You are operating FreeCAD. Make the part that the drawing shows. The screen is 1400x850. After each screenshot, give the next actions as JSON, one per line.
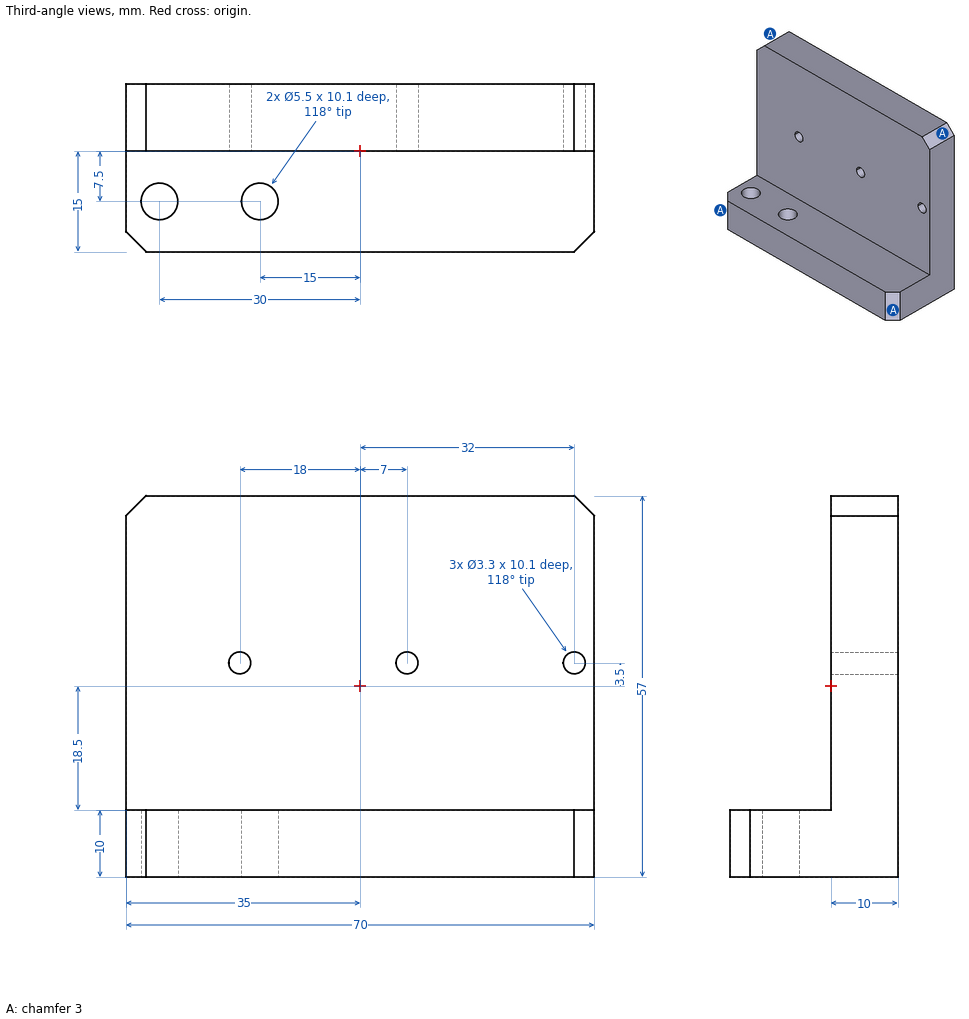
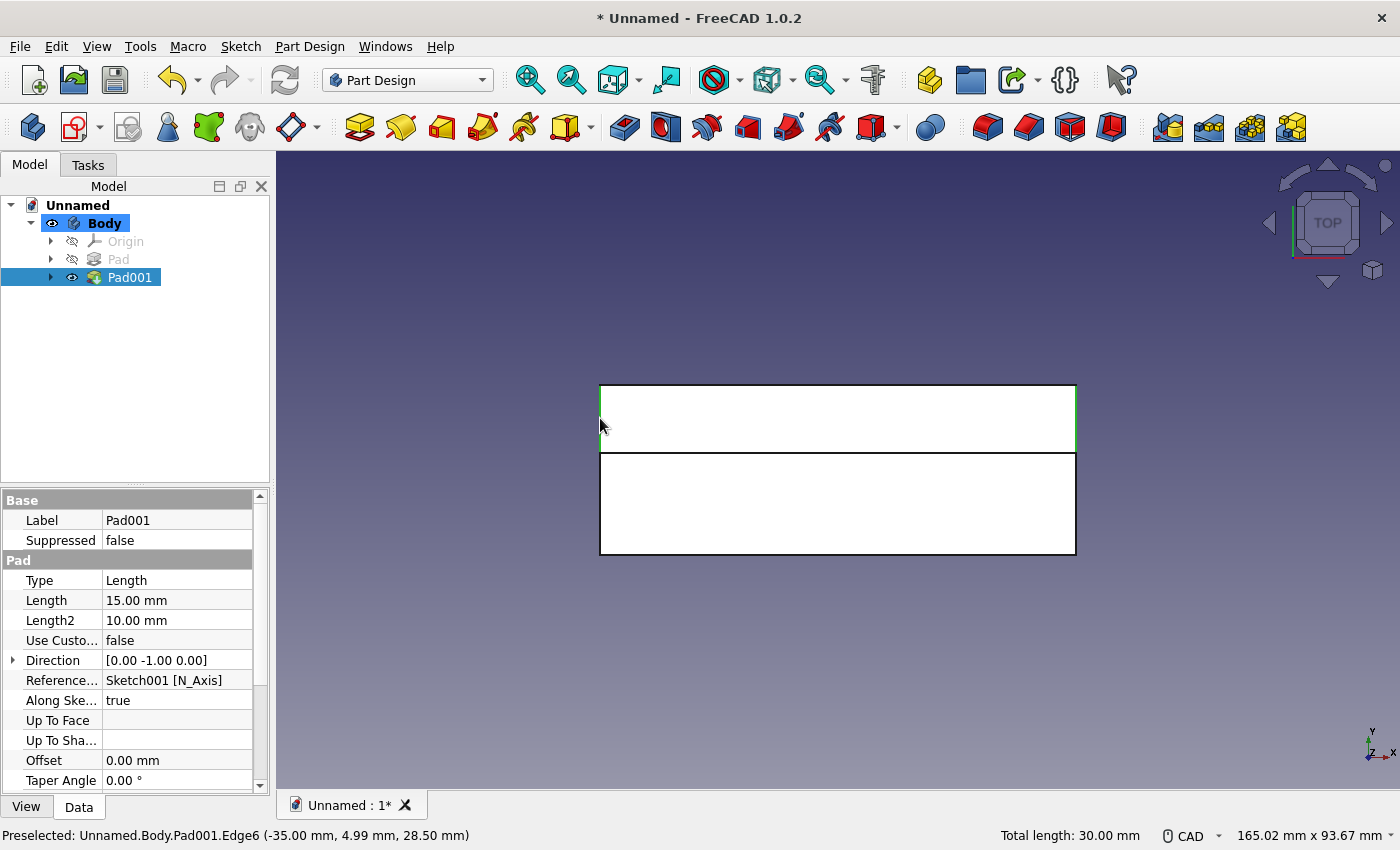
{"action": "key", "text": "1"}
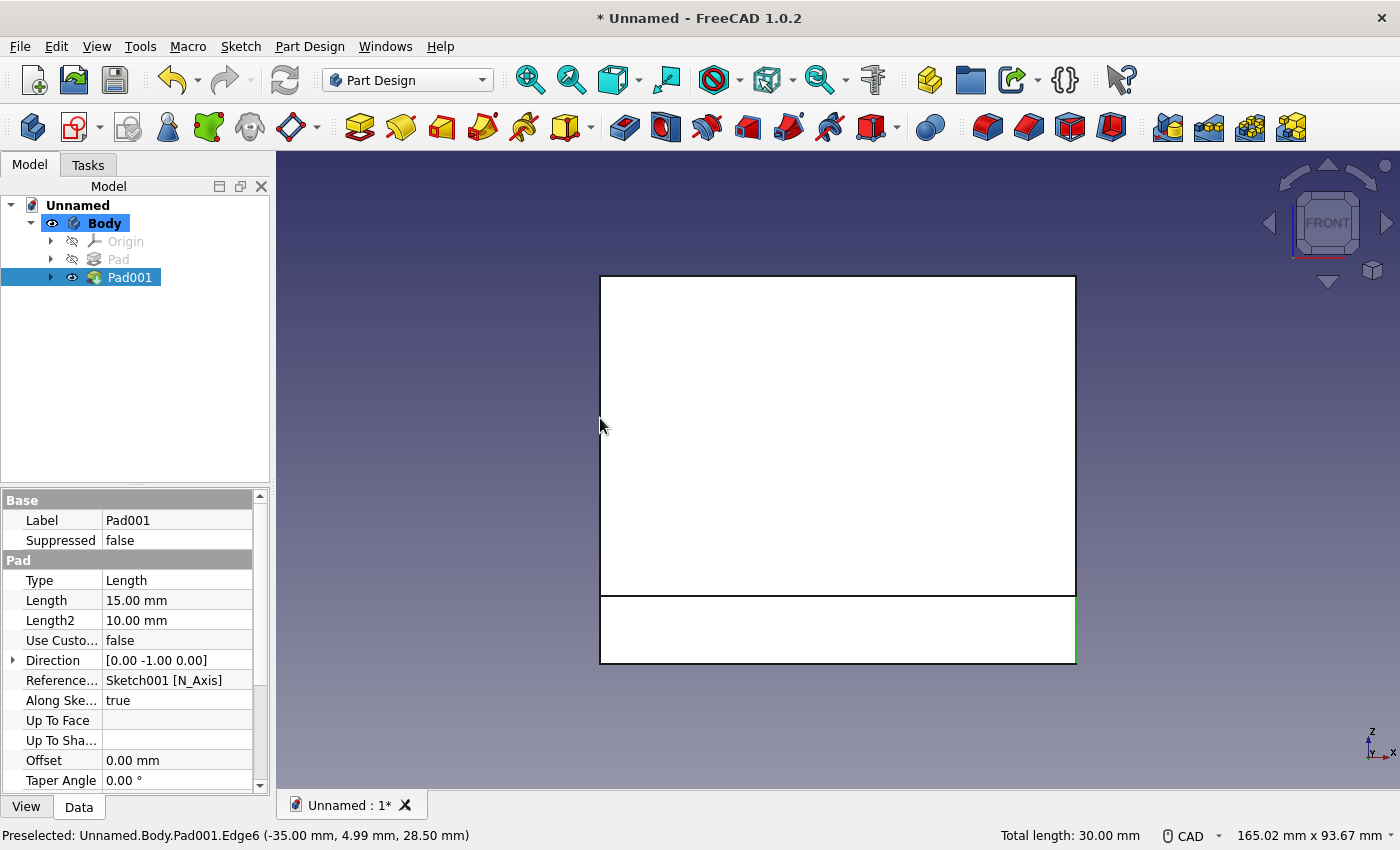
{"action": "left_click", "coordinate": [600, 629], "text": "ctrl"}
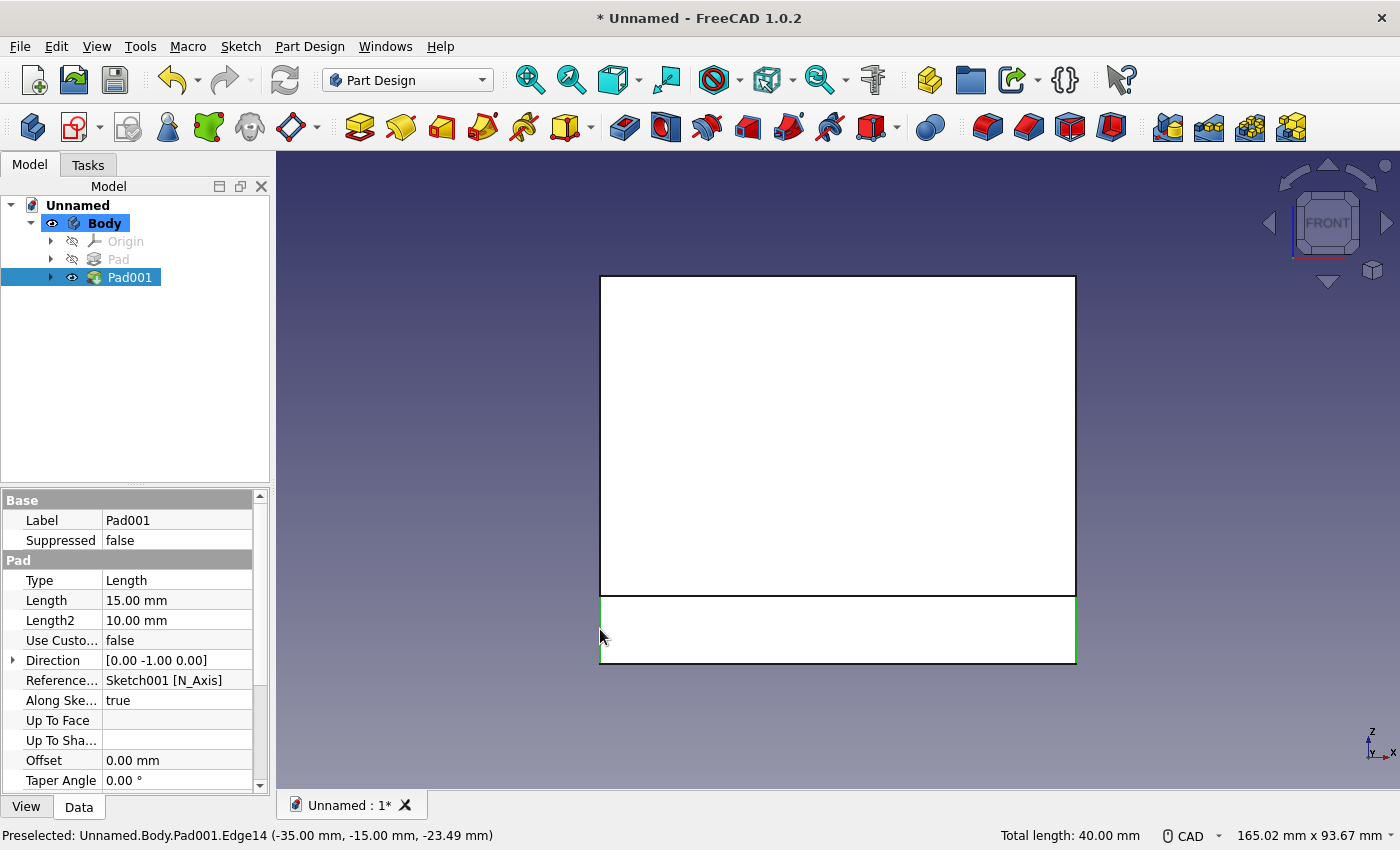
{"action": "left_click", "coordinate": [1029, 128]}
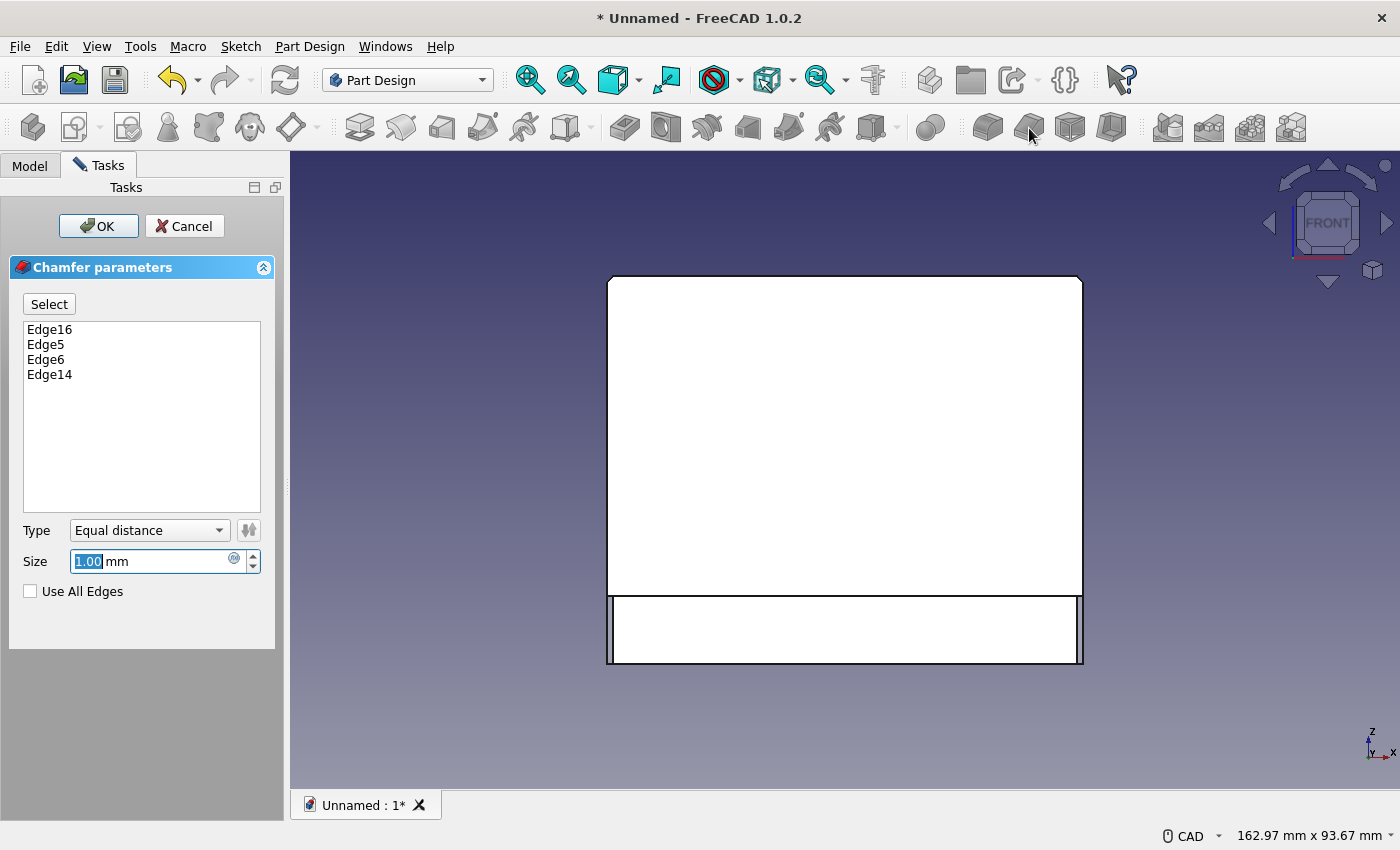
{"action": "type", "text": "3"}
{"action": "key", "text": "Tab"}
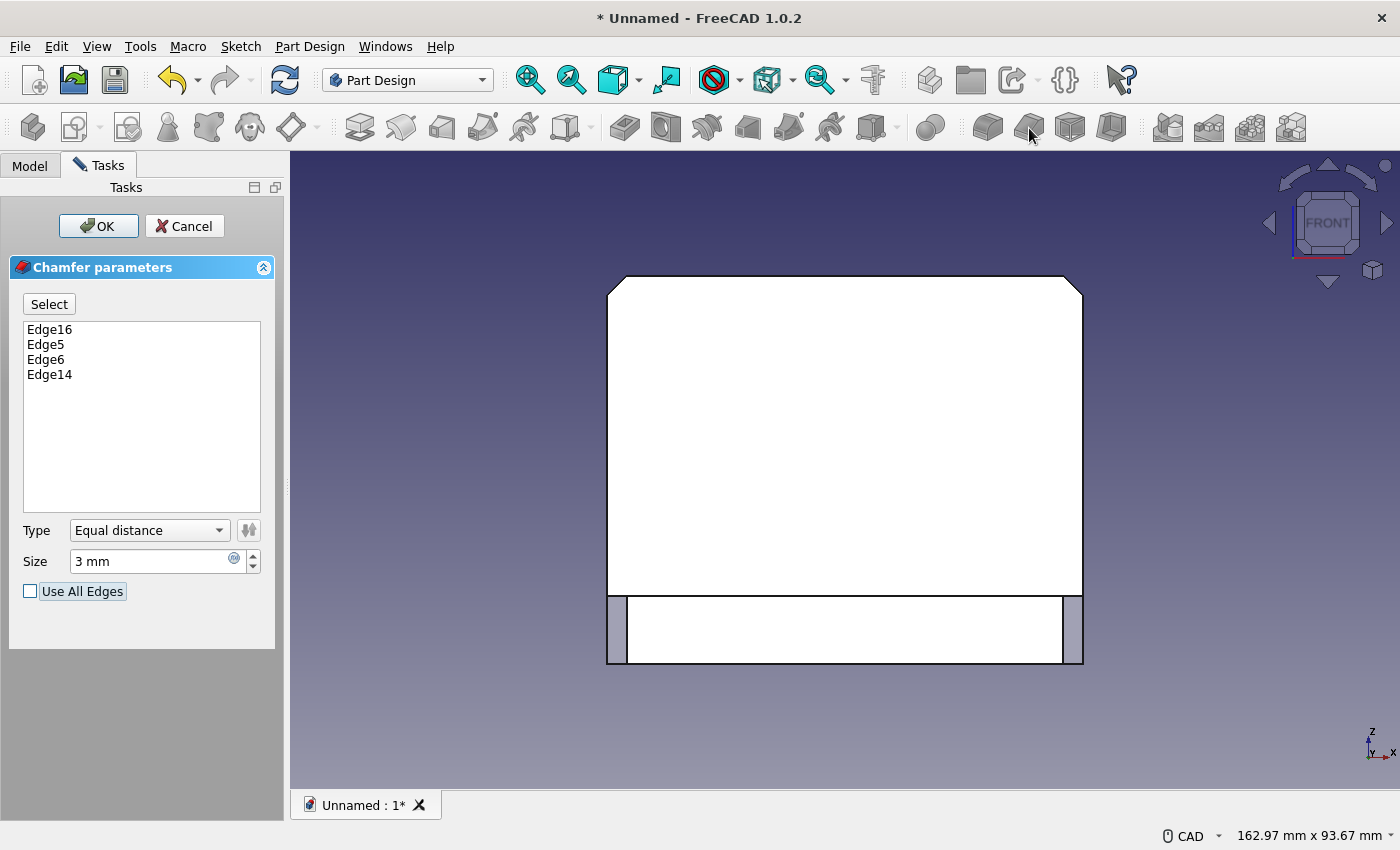
{"action": "left_click", "coordinate": [99, 226]}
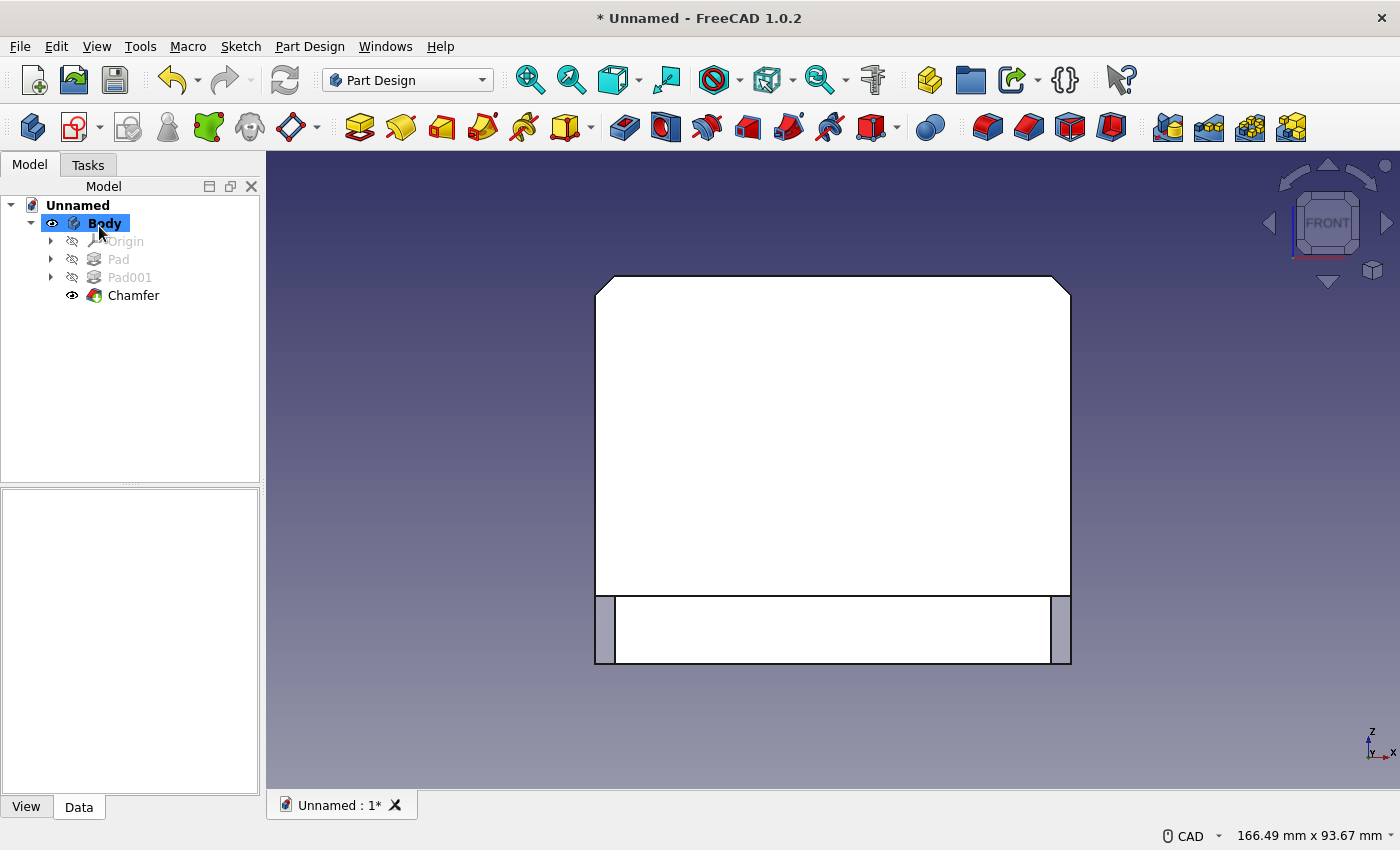
{"action": "key", "text": "4"}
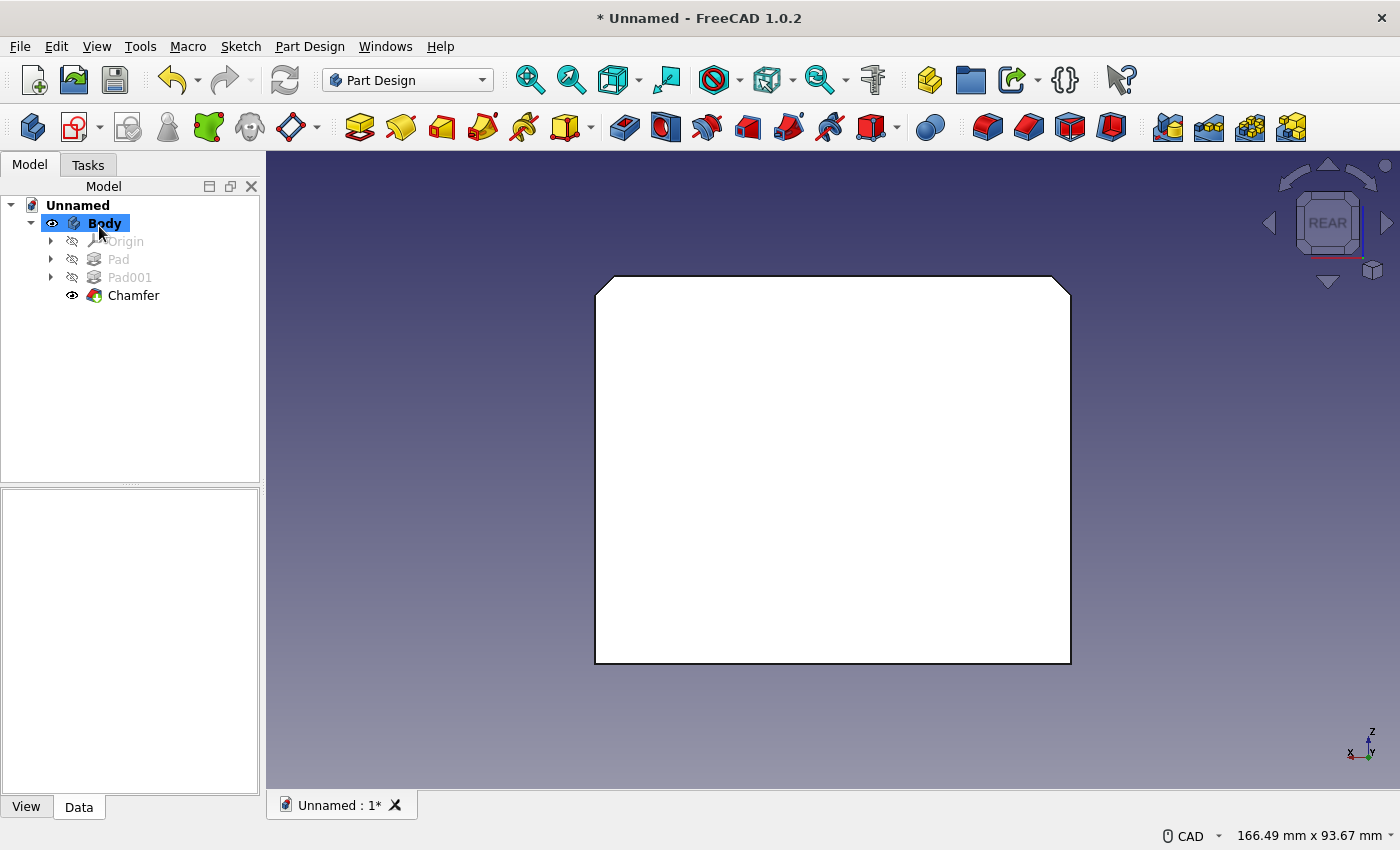
{"action": "left_click", "coordinate": [833, 469]}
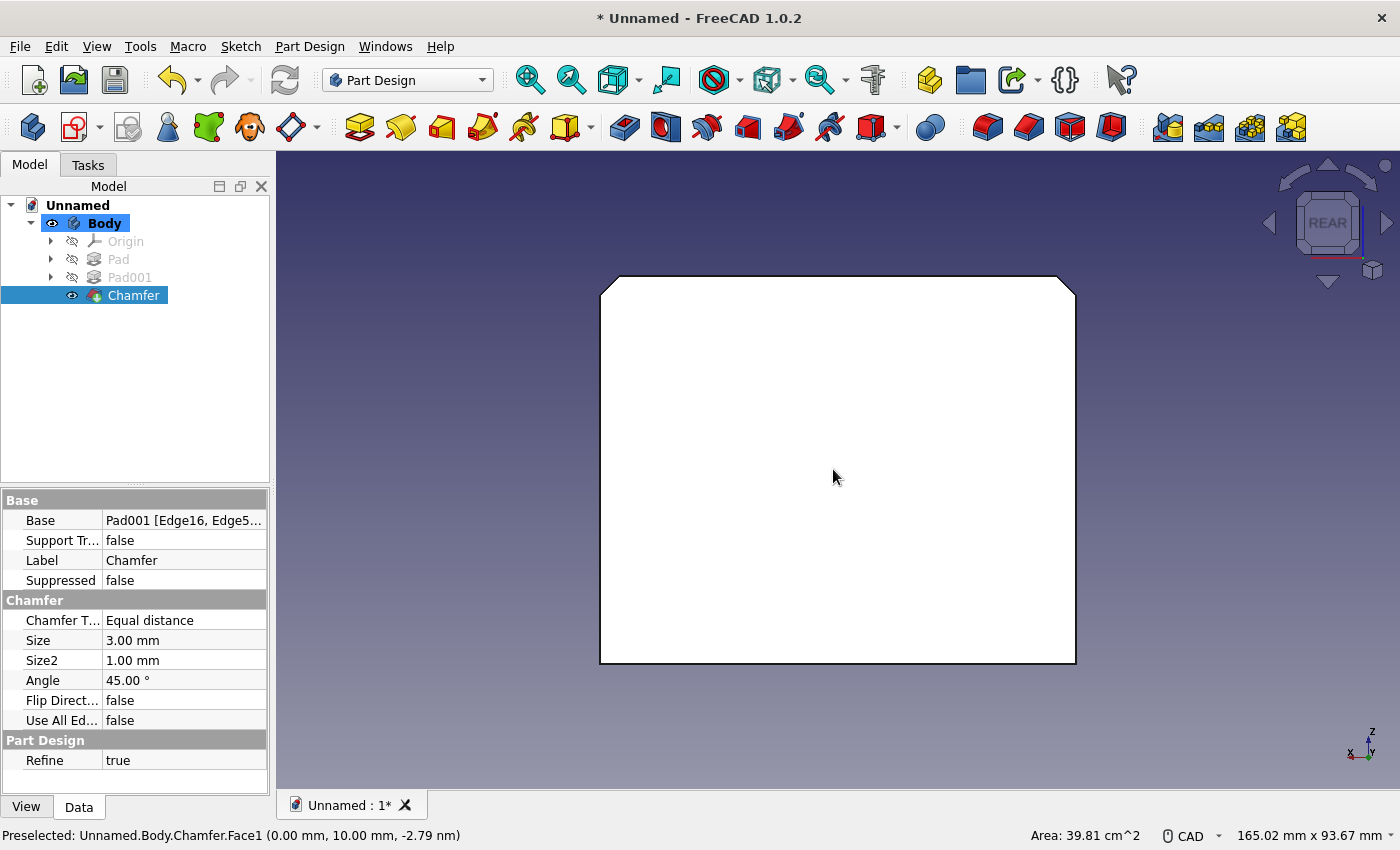
{"action": "left_click", "coordinate": [74, 128]}